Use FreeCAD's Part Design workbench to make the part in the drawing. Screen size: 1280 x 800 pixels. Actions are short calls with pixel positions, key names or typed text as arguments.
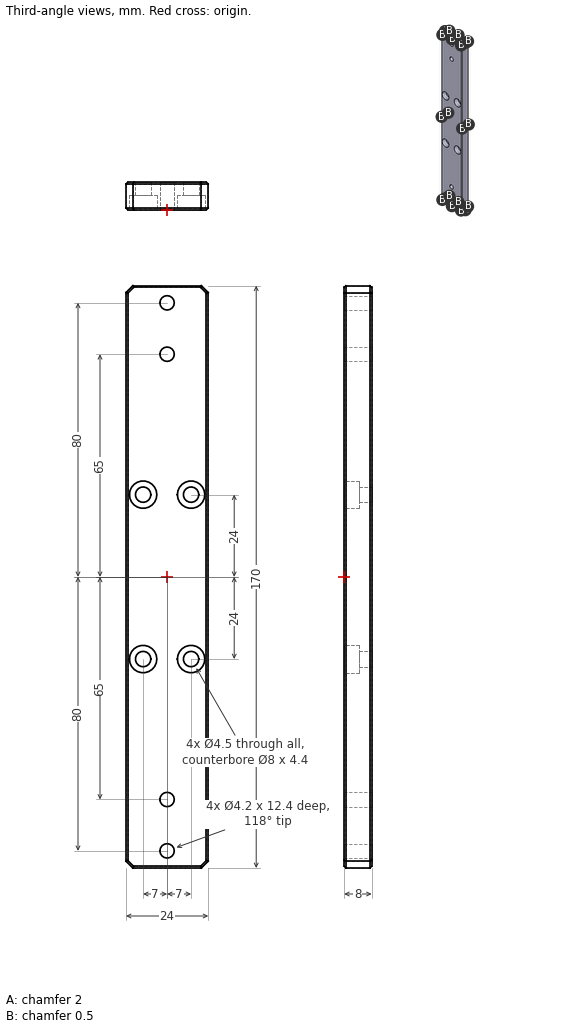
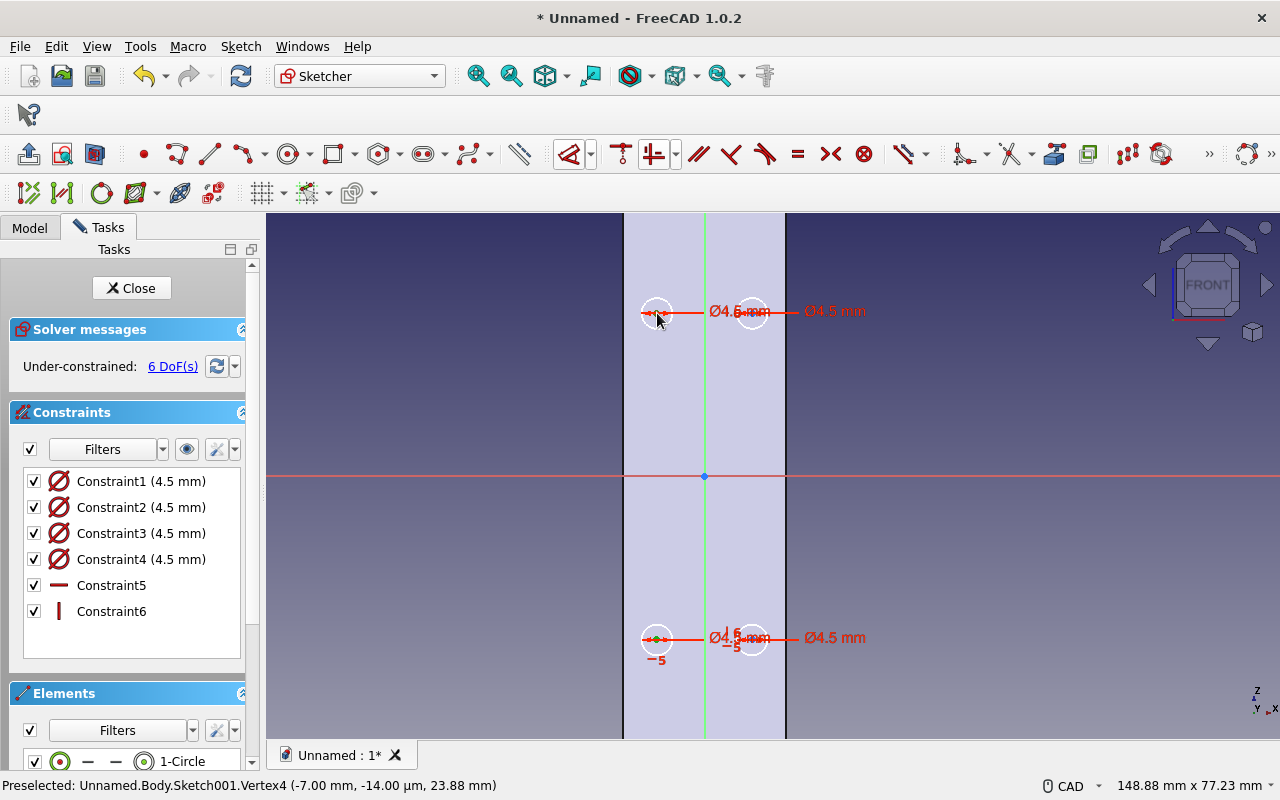
key(v)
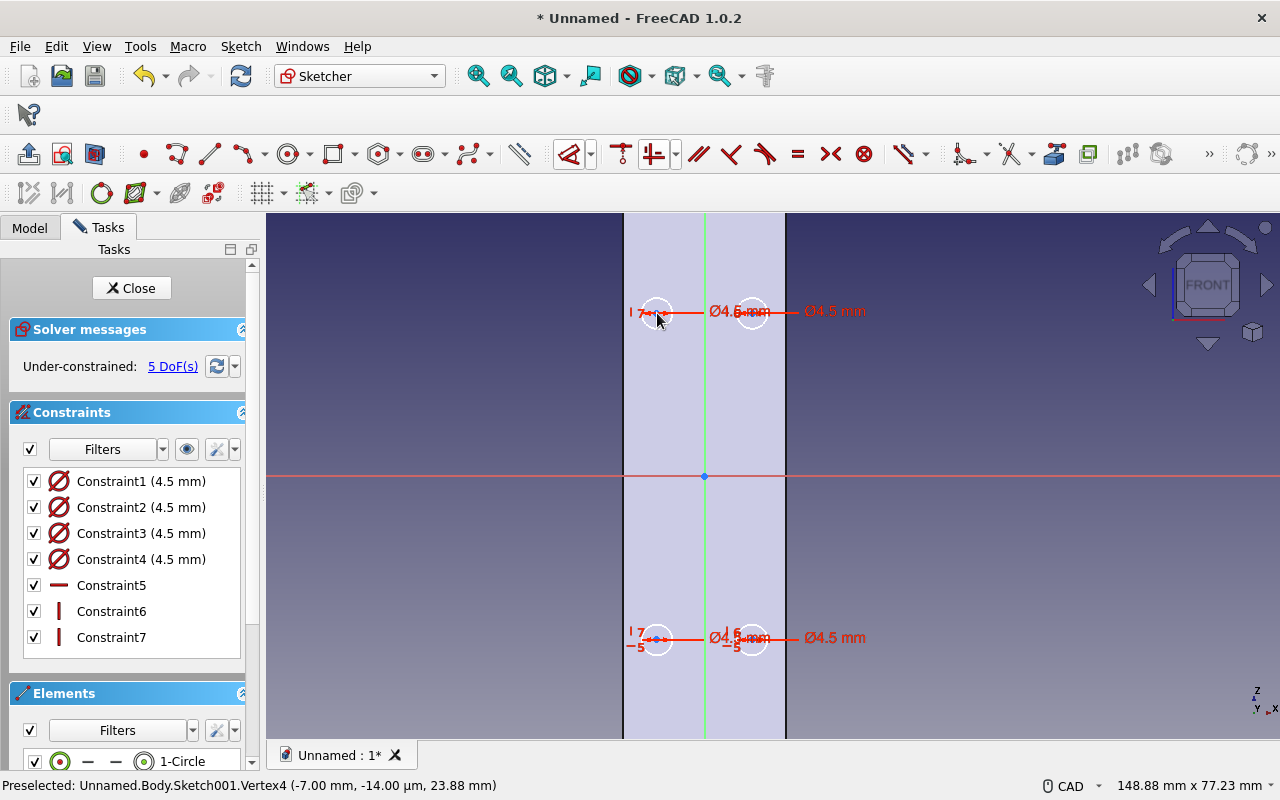
click(752, 313)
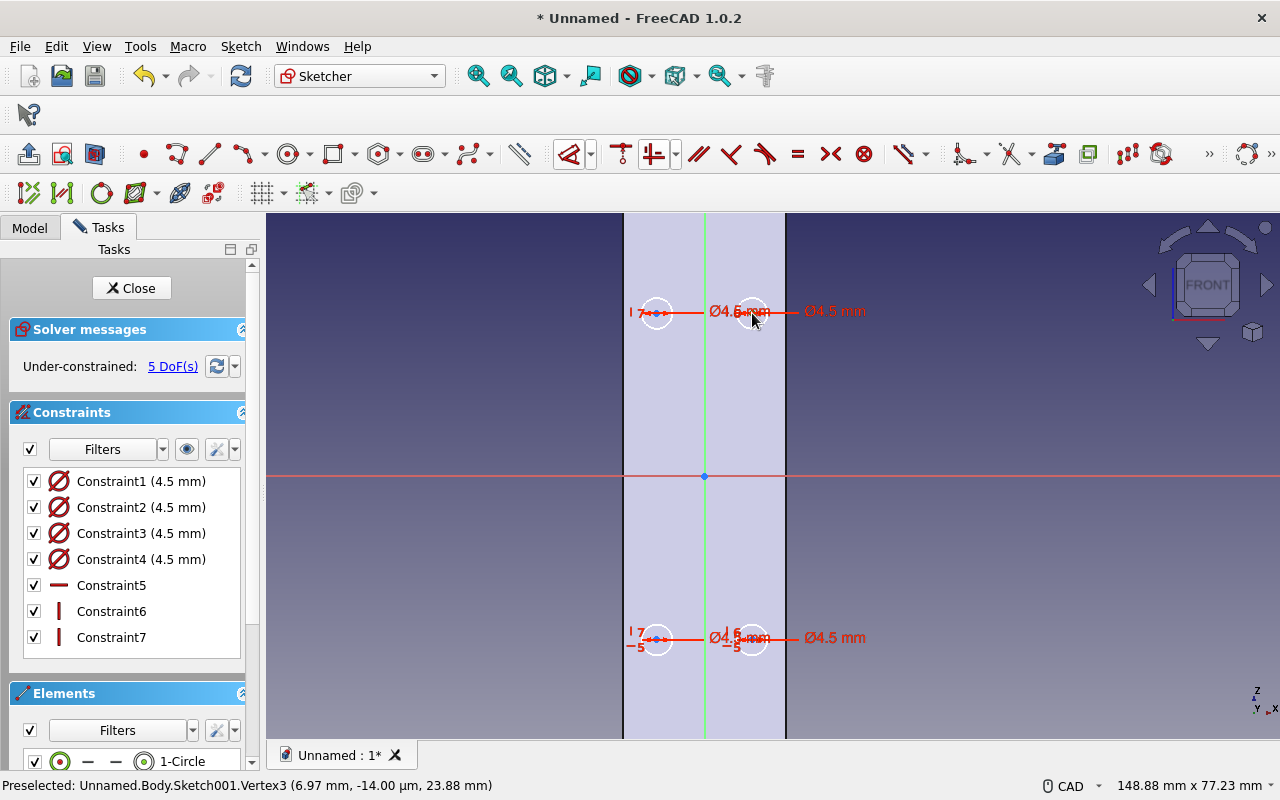
click(657, 313)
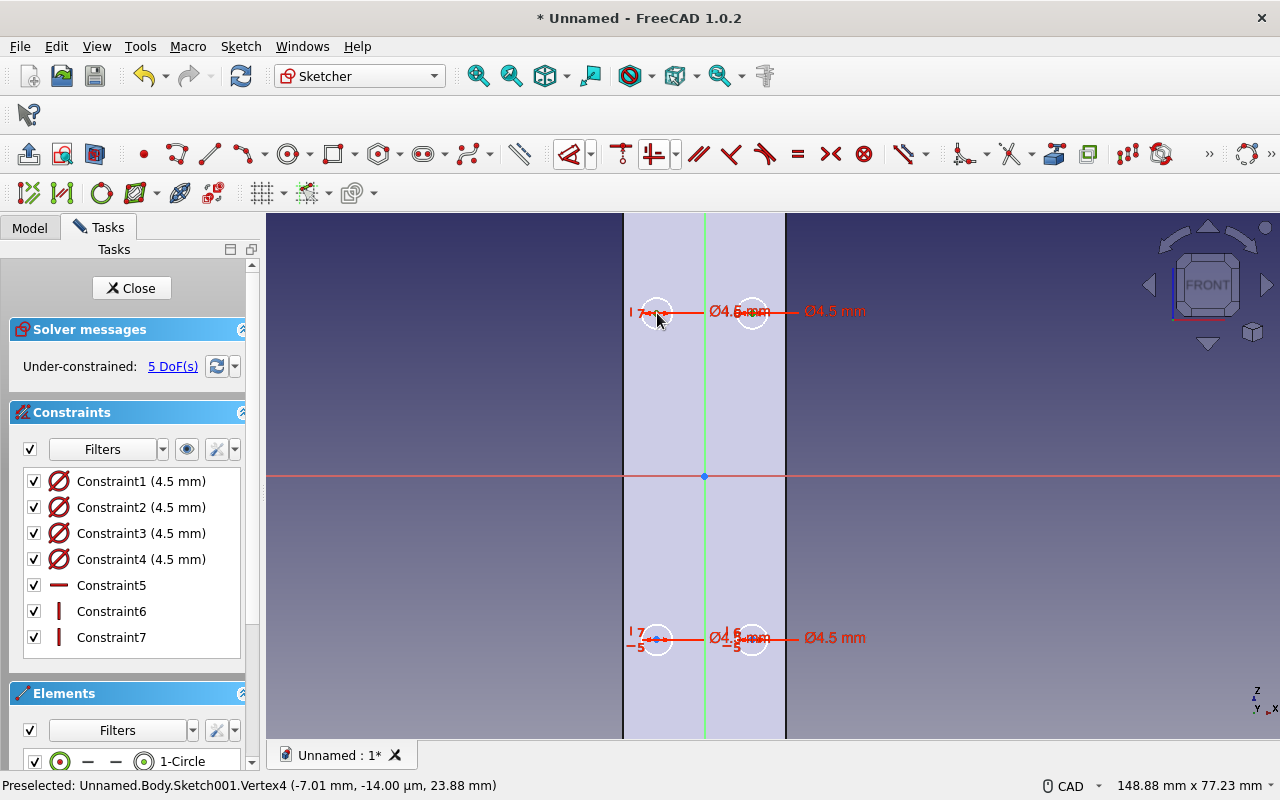
key(h)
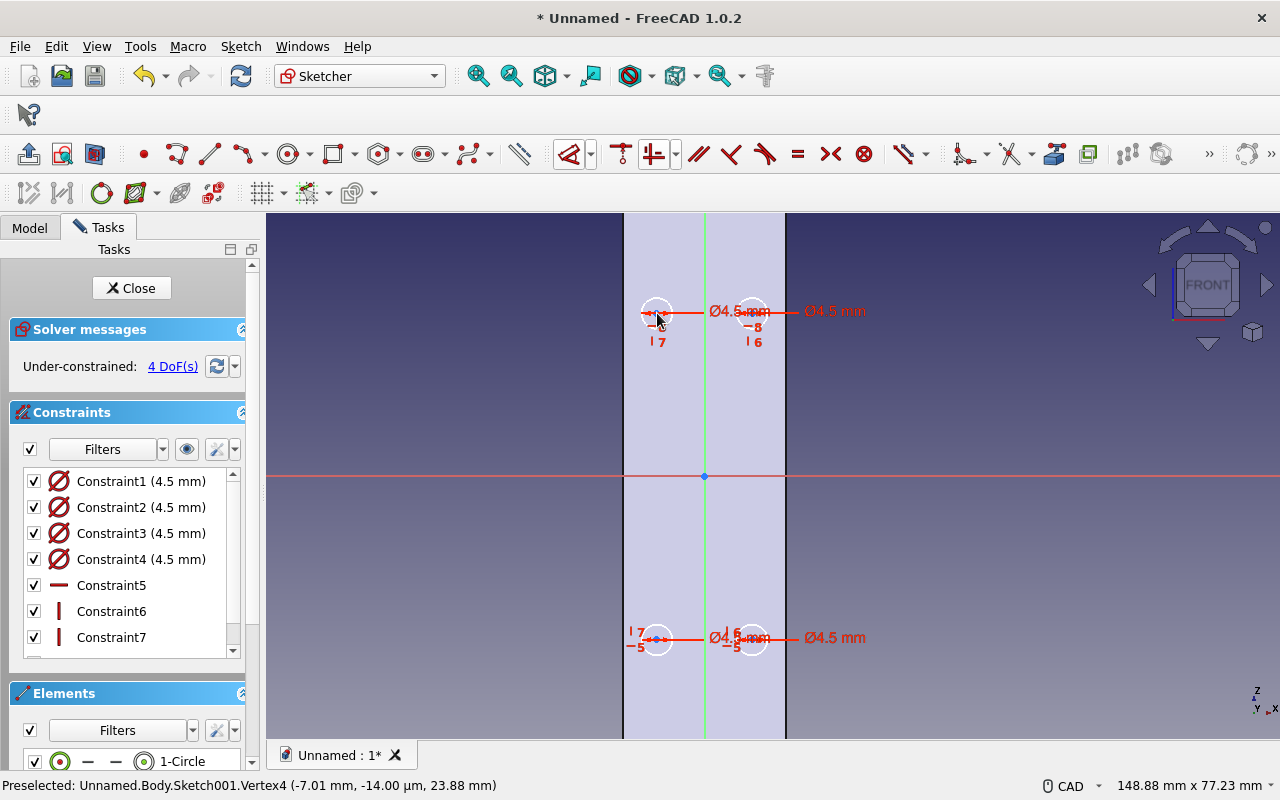
click(752, 640)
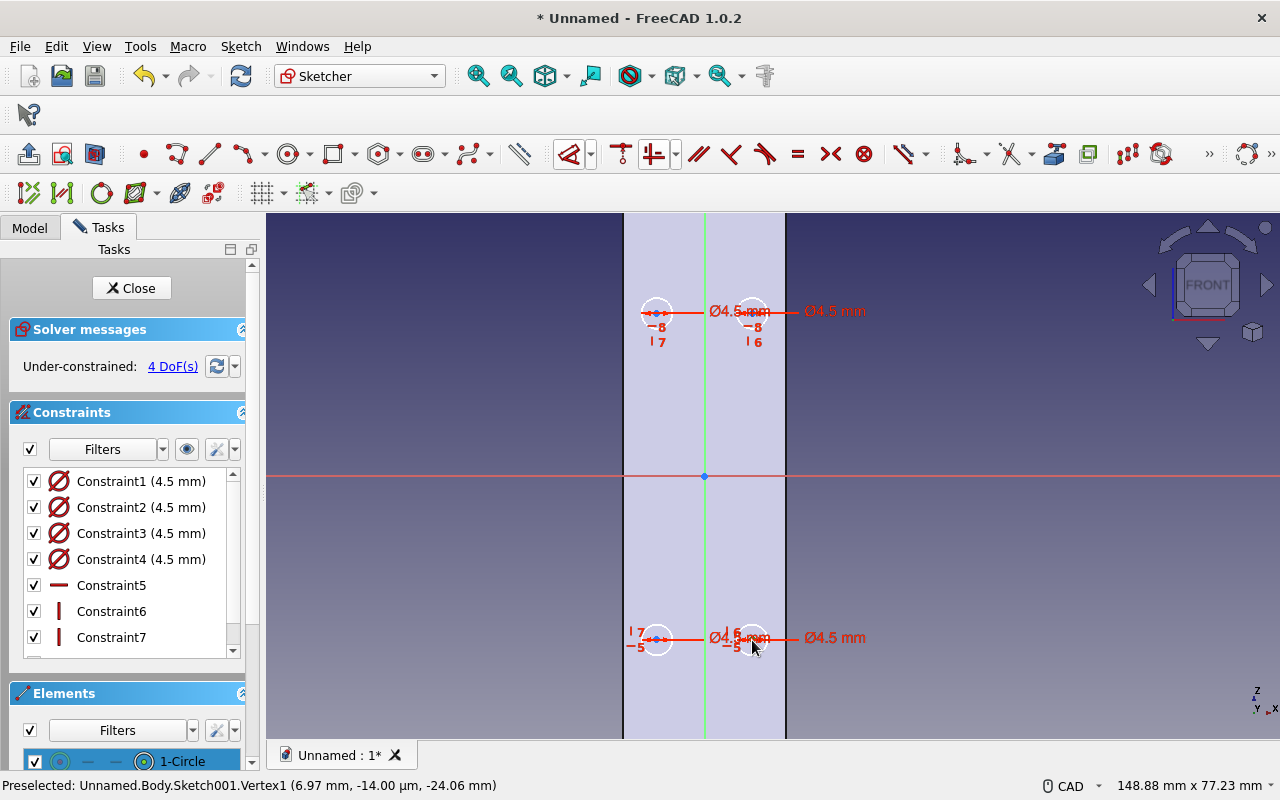
click(590, 154)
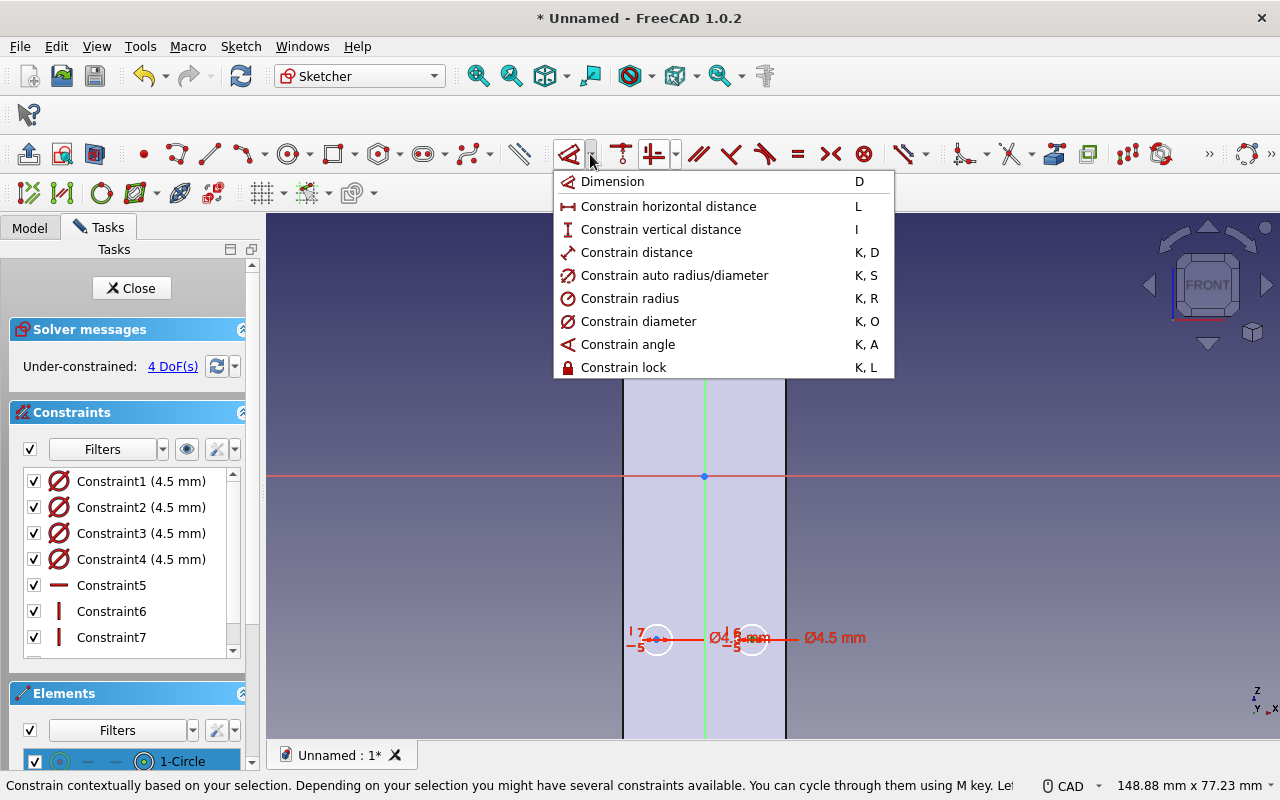
click(724, 206)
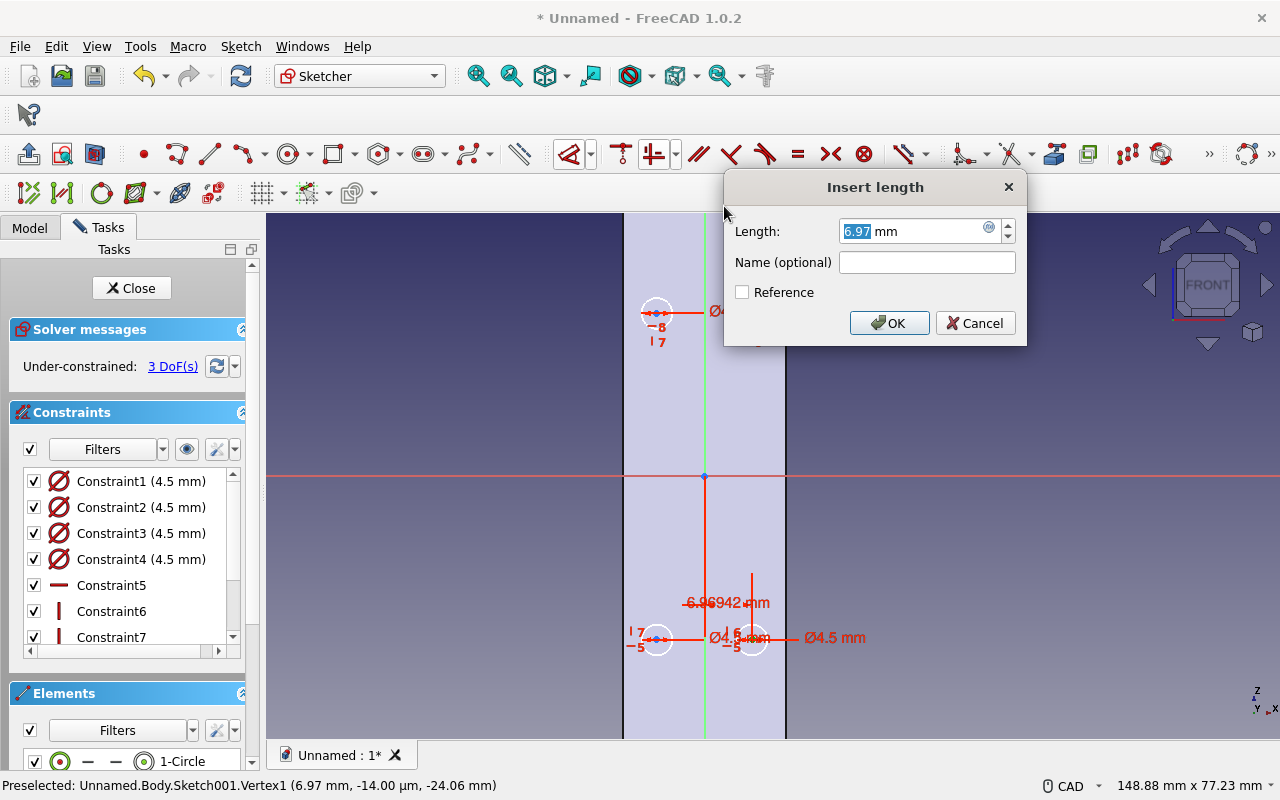
text(7)
key(Return)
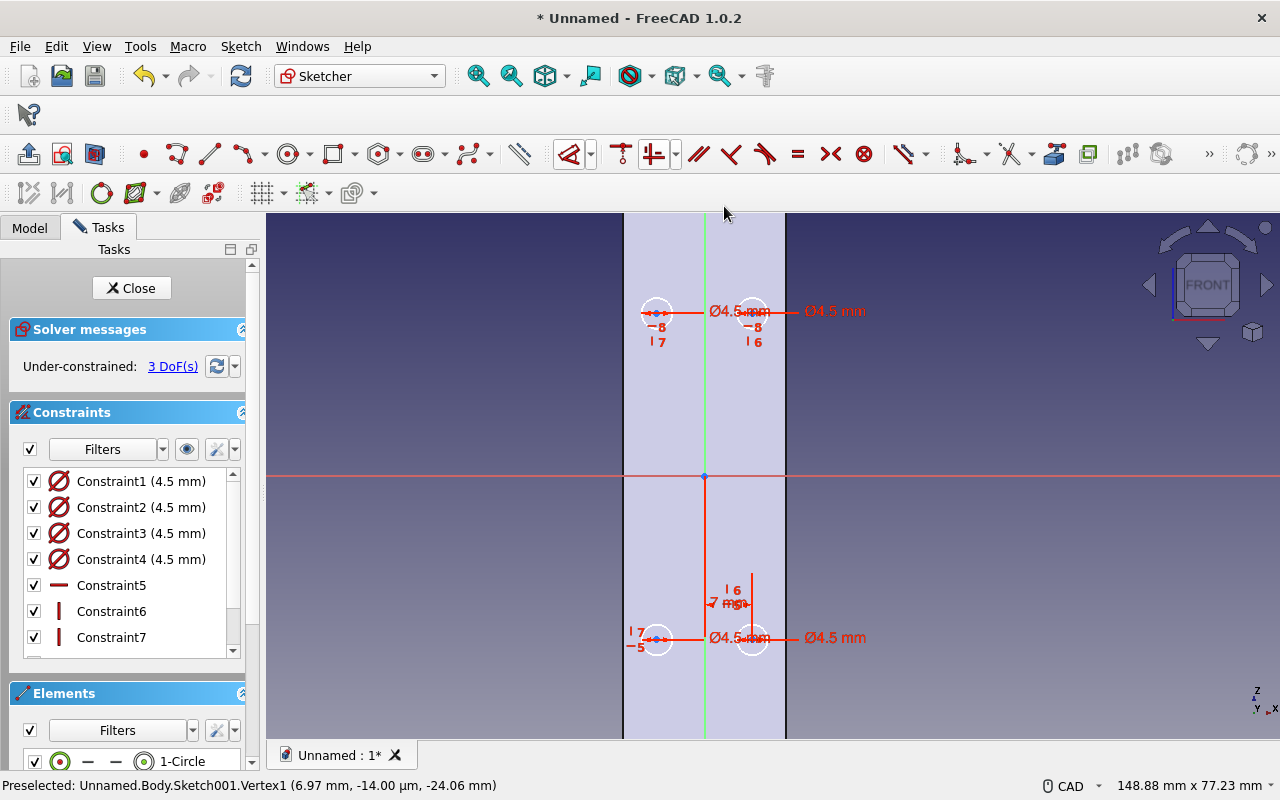
click(657, 640)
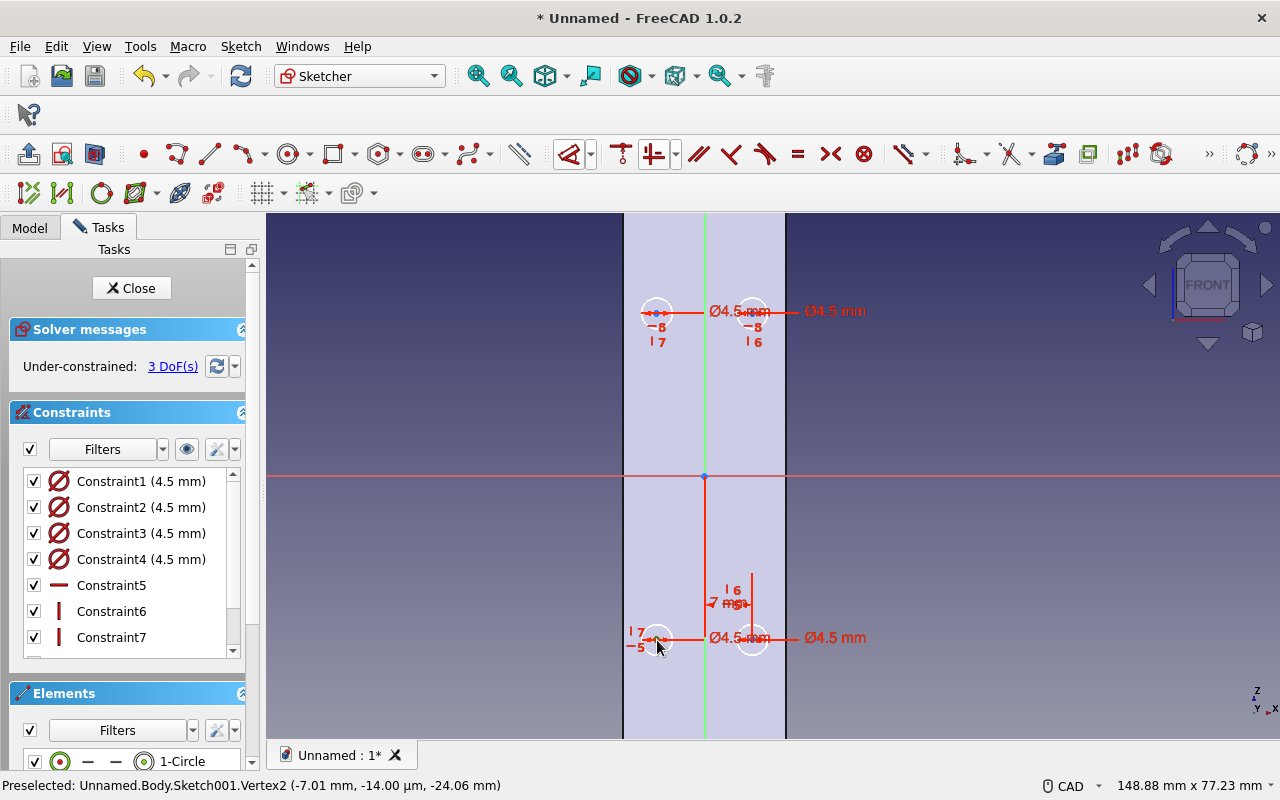
key(l)